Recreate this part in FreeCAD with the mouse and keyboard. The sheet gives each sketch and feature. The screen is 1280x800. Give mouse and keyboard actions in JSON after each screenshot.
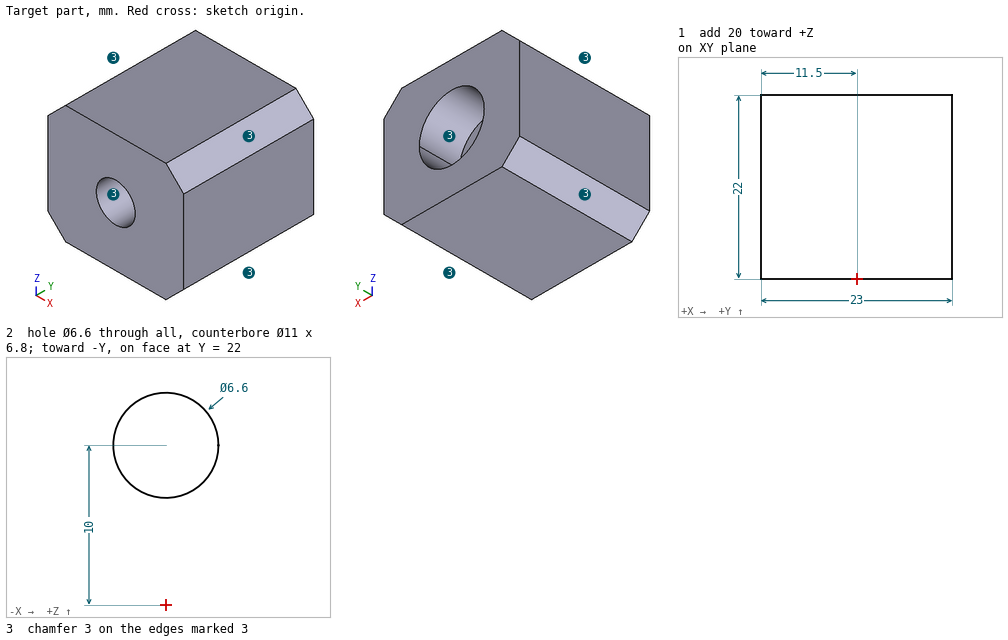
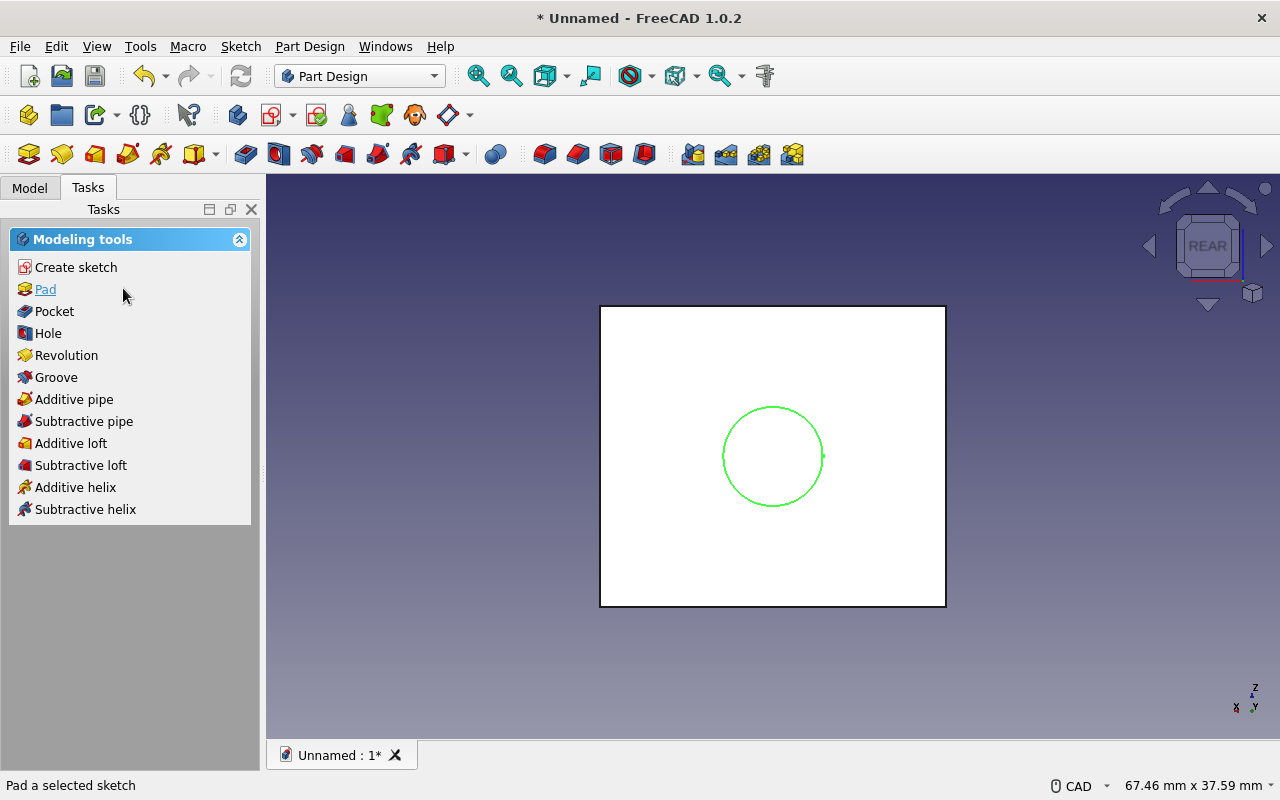
{"action": "left_click", "coordinate": [279, 154]}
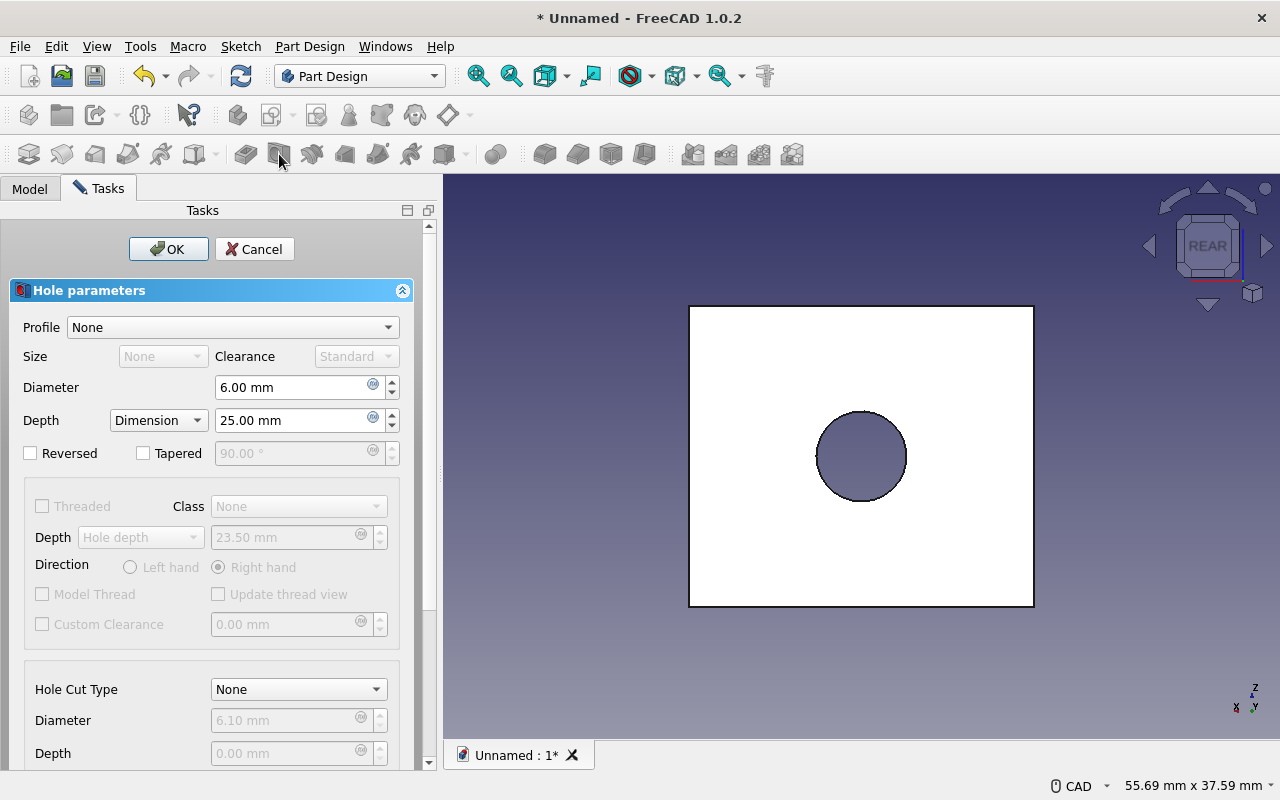
{"action": "triple_click", "coordinate": [300, 388]}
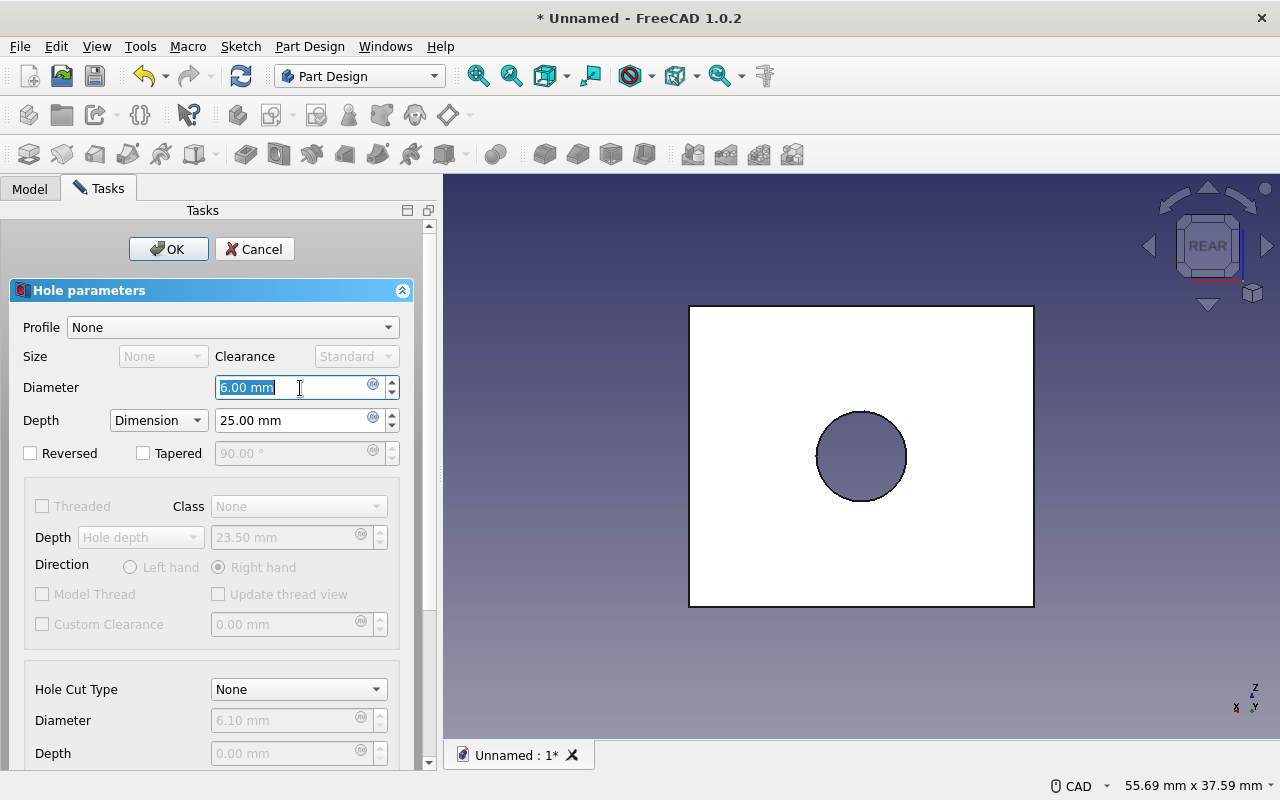
{"action": "type", "text": "6.6"}
{"action": "key", "text": "Tab"}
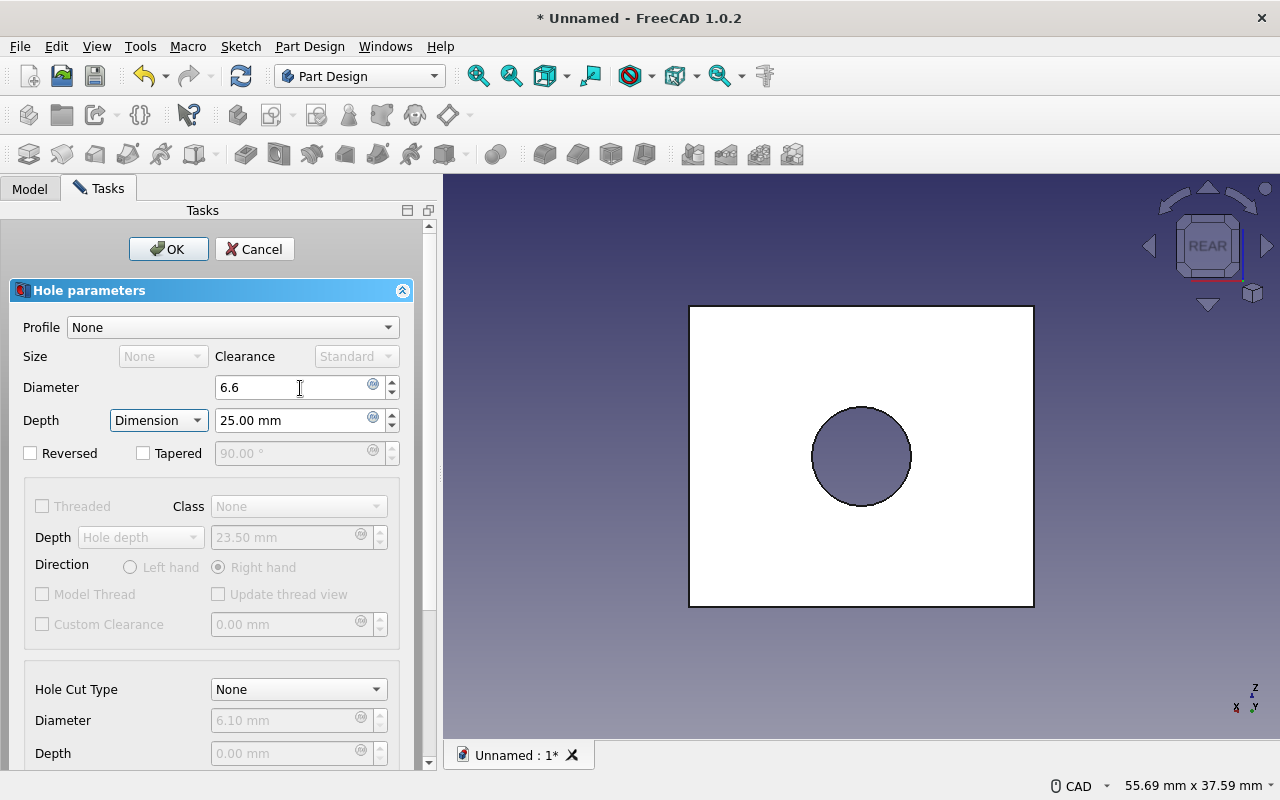
{"action": "left_click", "coordinate": [160, 420]}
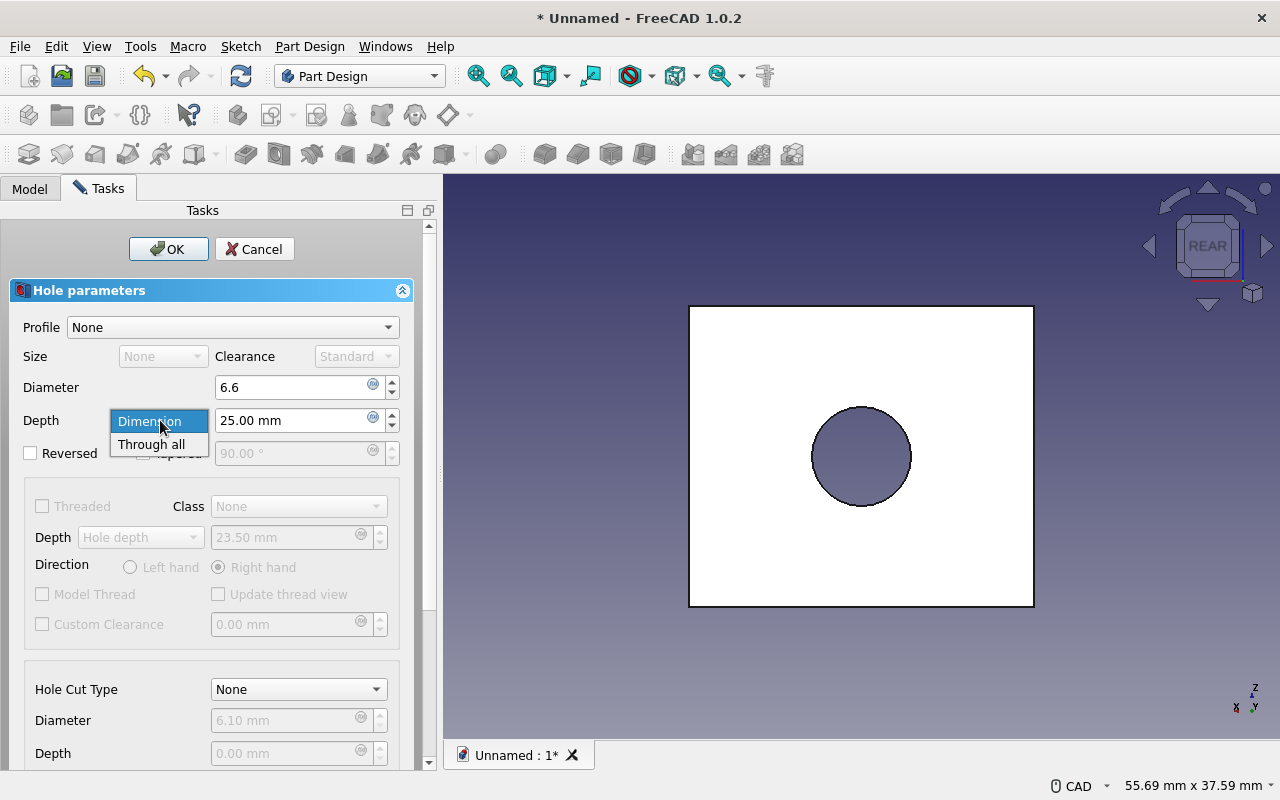
{"action": "left_click", "coordinate": [158, 444]}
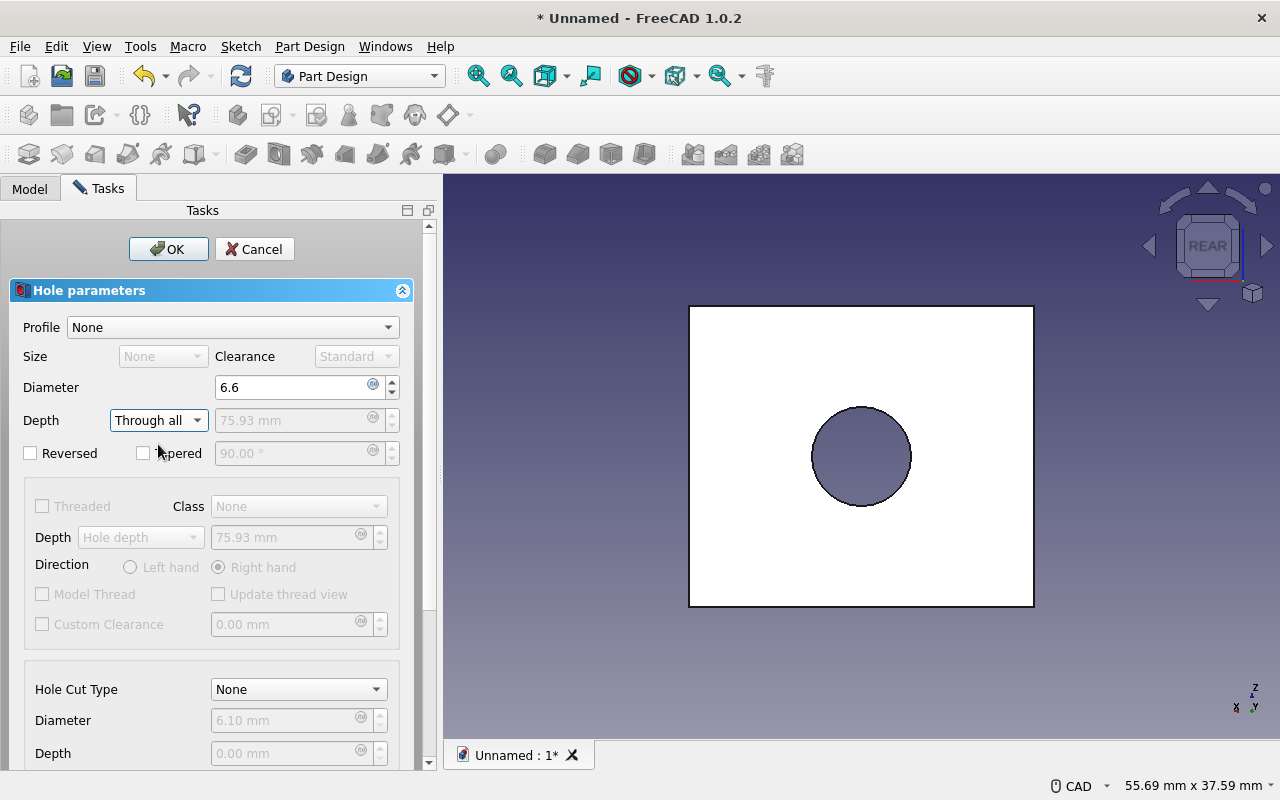
{"action": "left_click", "coordinate": [300, 690]}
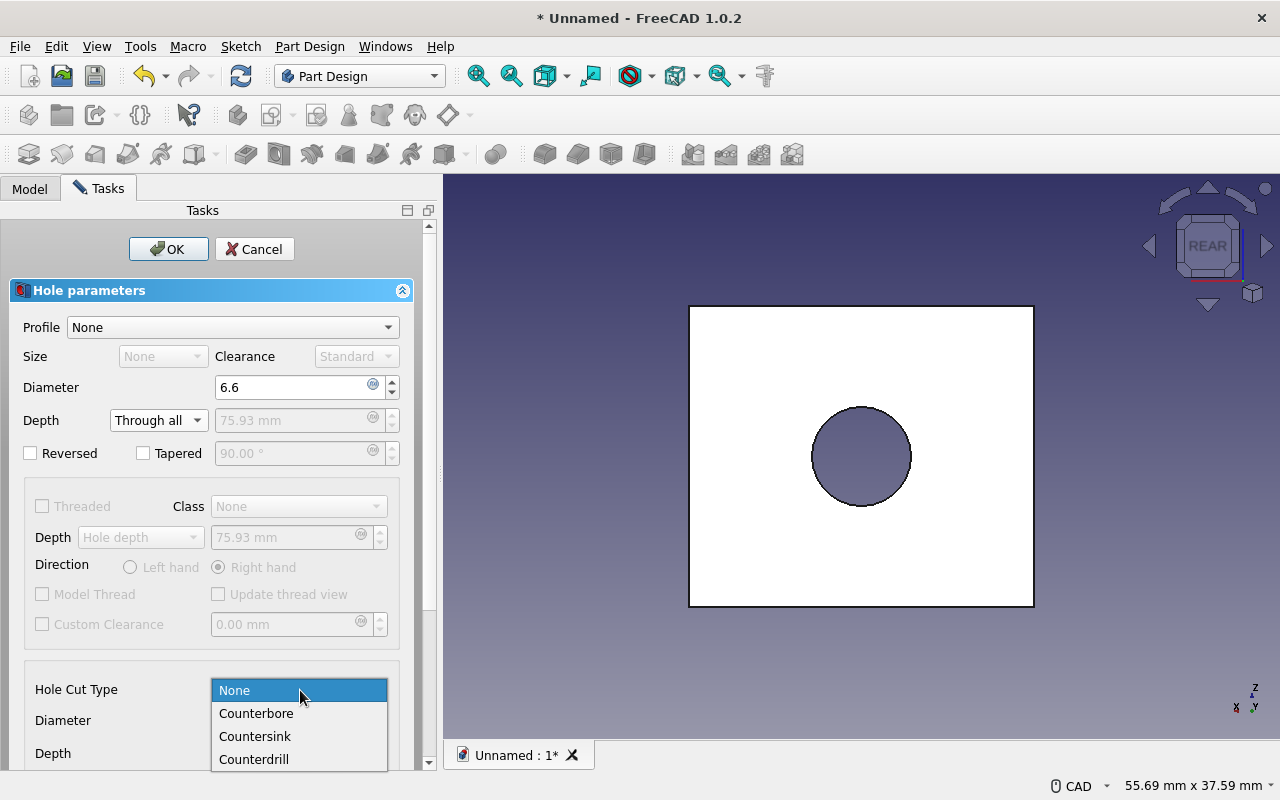
{"action": "left_click", "coordinate": [298, 714]}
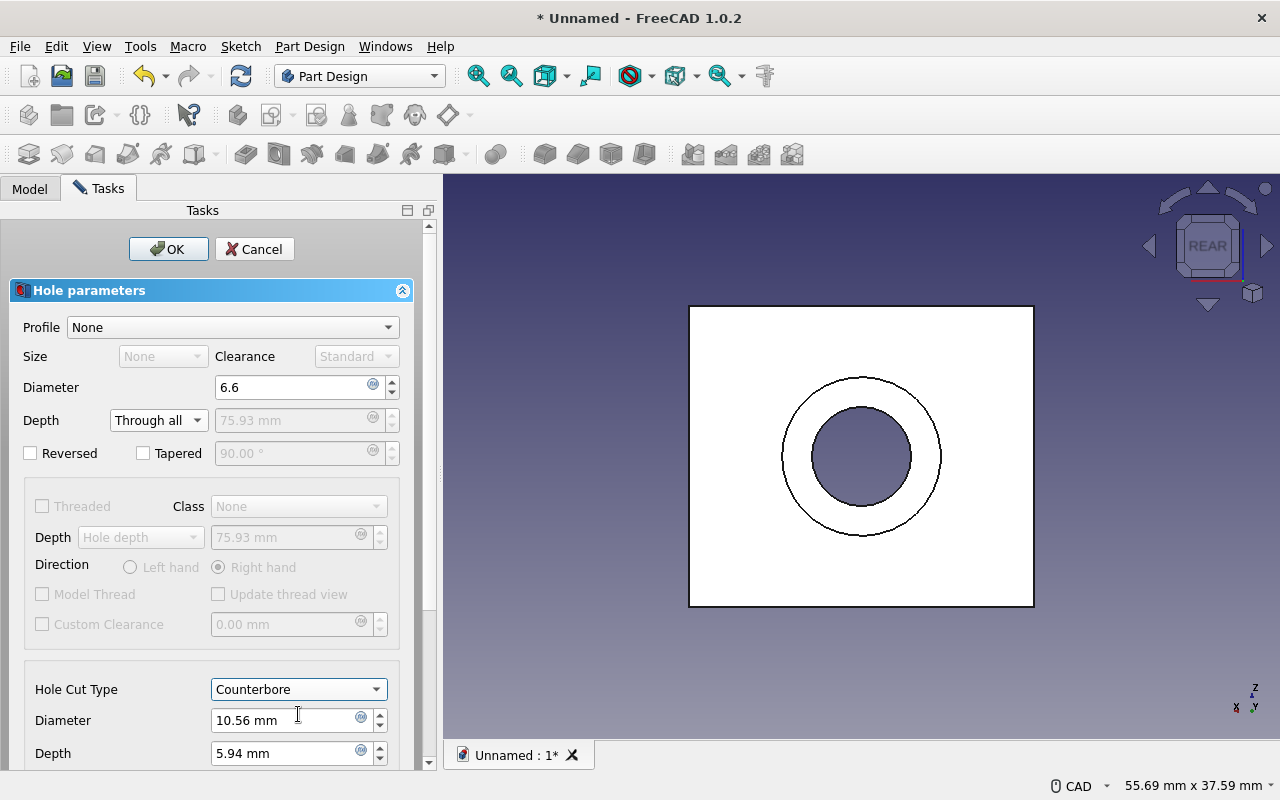
{"action": "triple_click", "coordinate": [292, 720]}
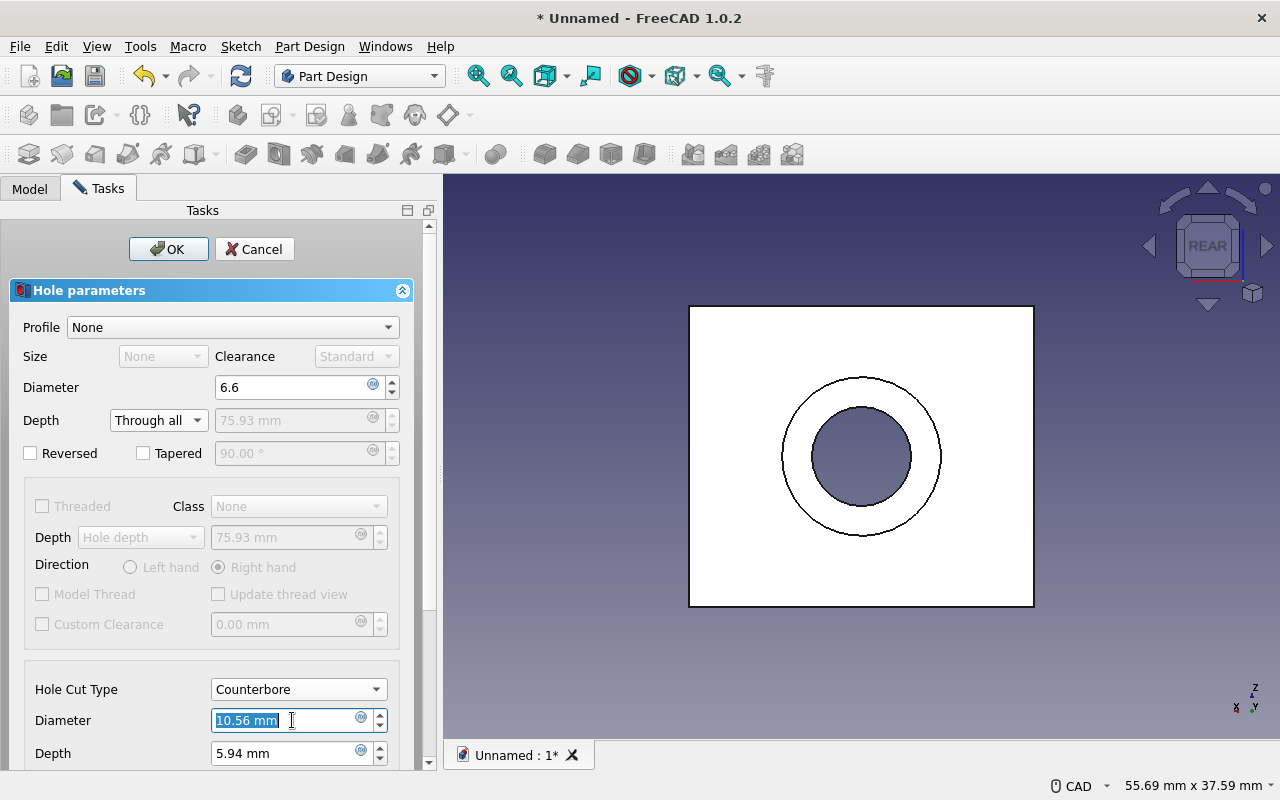
{"action": "type", "text": "11"}
{"action": "key", "text": "Tab"}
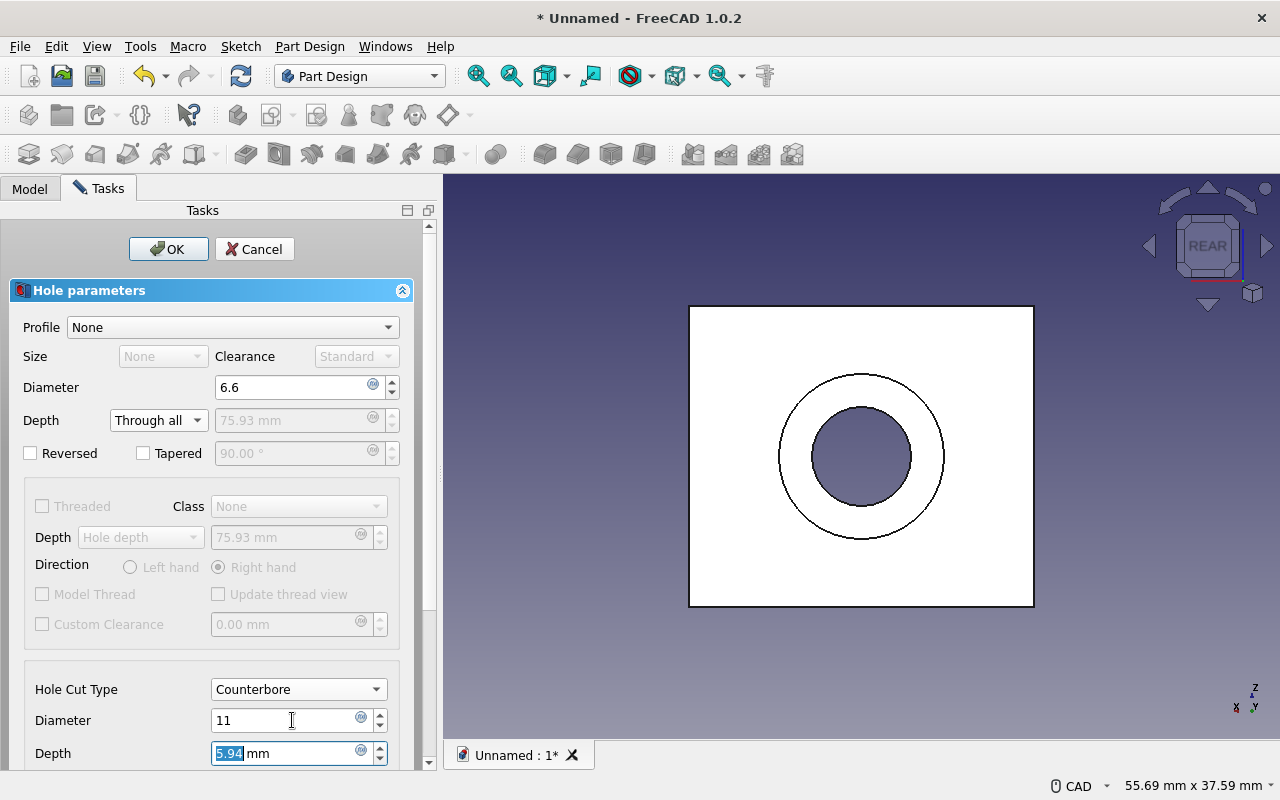
{"action": "type", "text": "6.8"}
{"action": "key", "text": "Tab"}